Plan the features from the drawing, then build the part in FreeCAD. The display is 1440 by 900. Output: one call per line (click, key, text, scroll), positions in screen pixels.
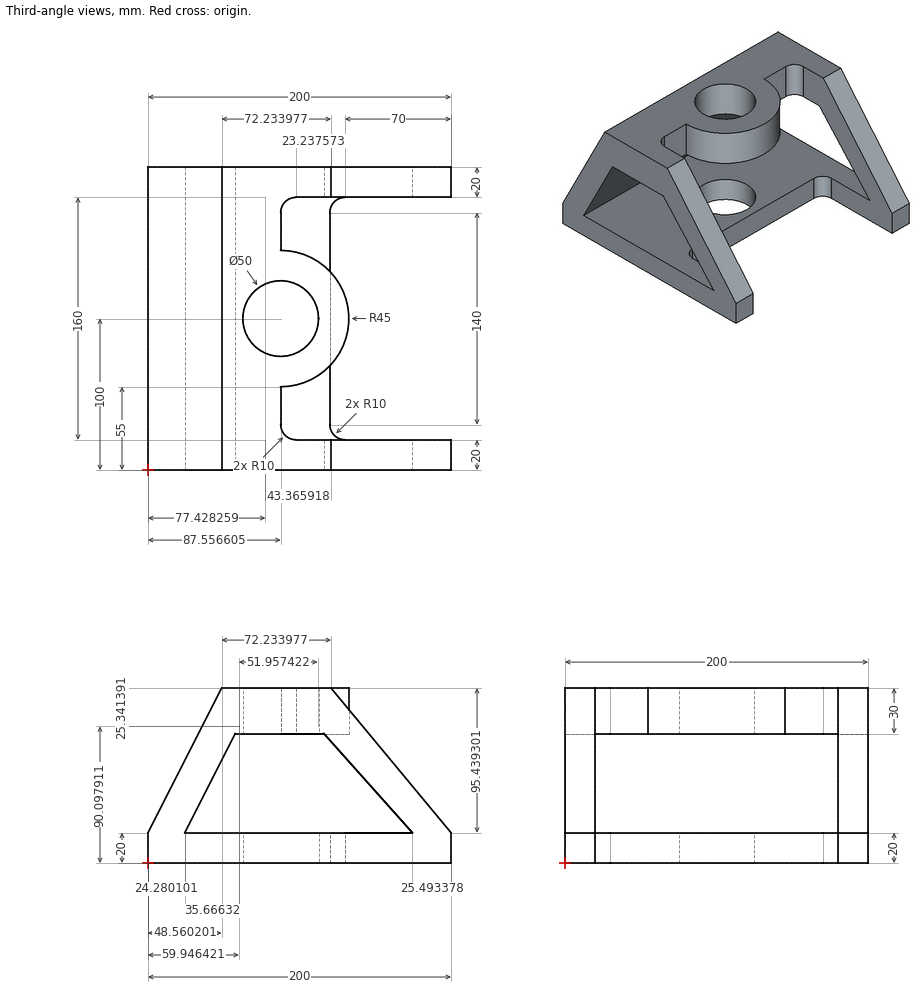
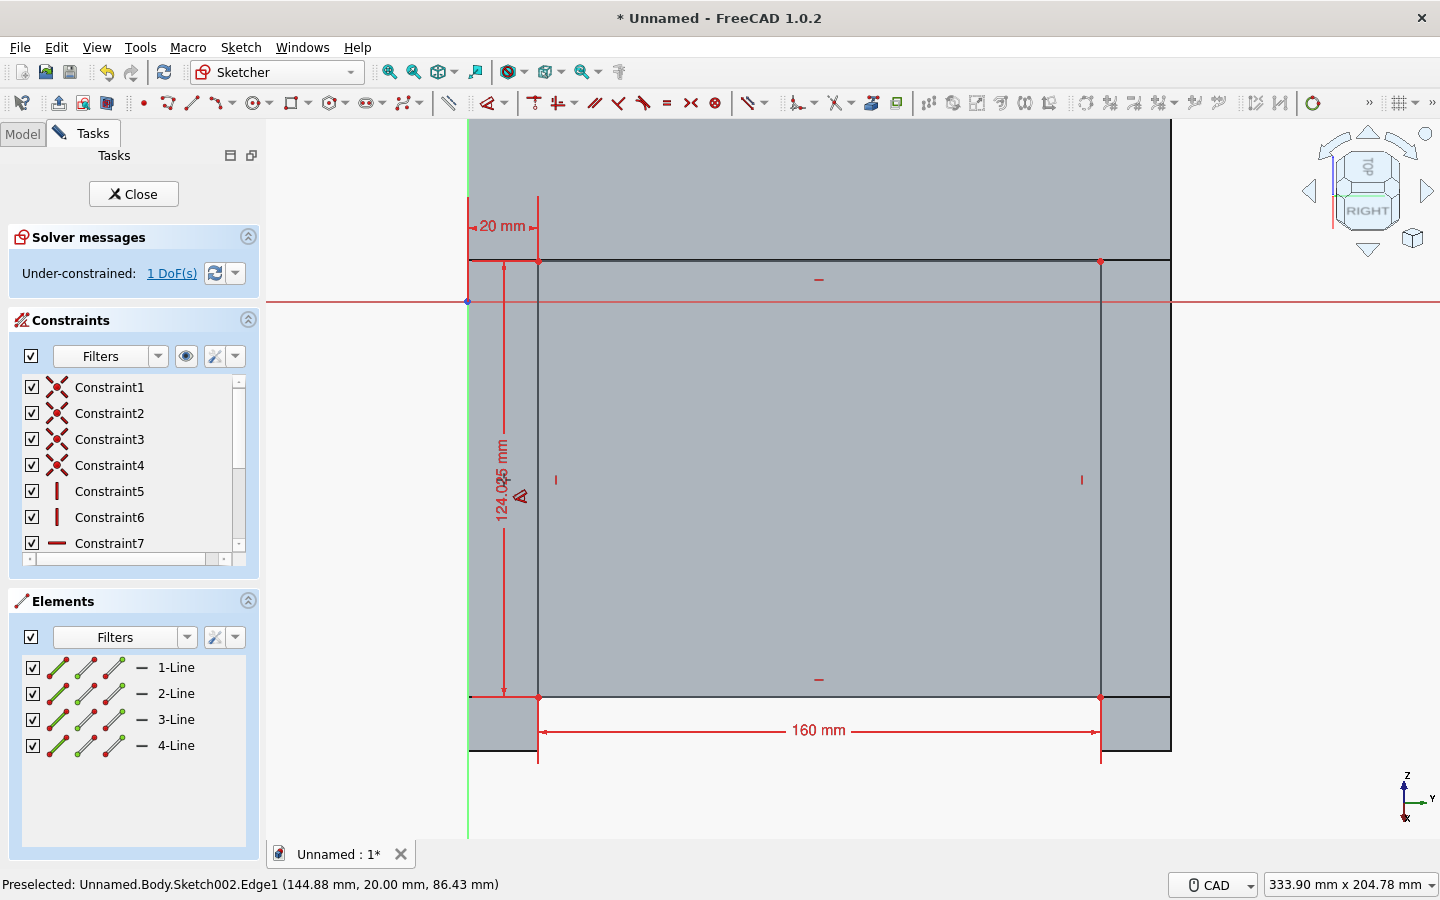
click(538, 261)
click(434, 281)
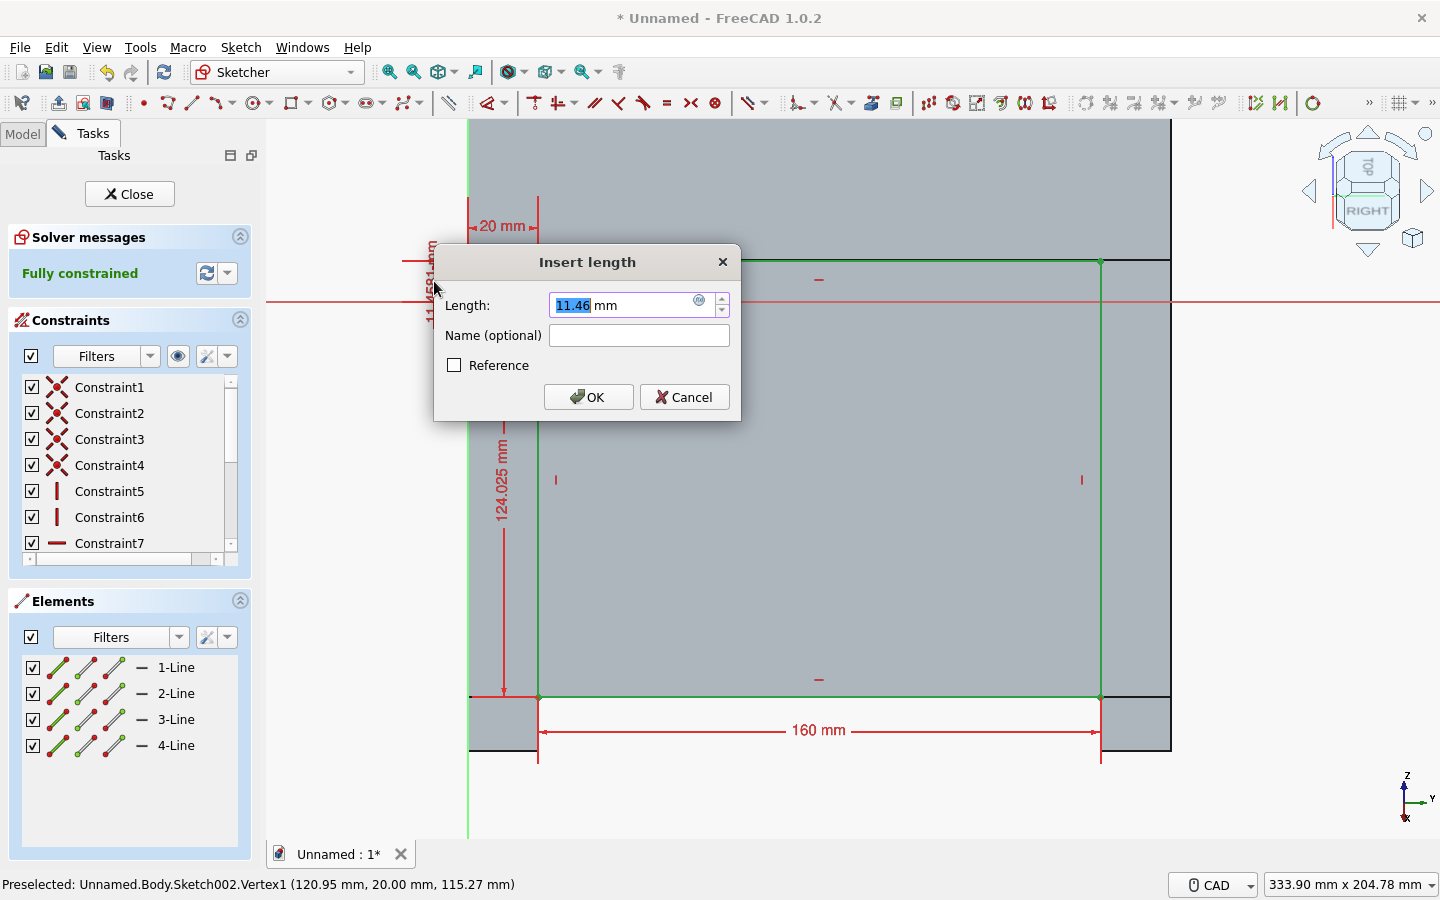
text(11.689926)
key(Return)
key(Escape)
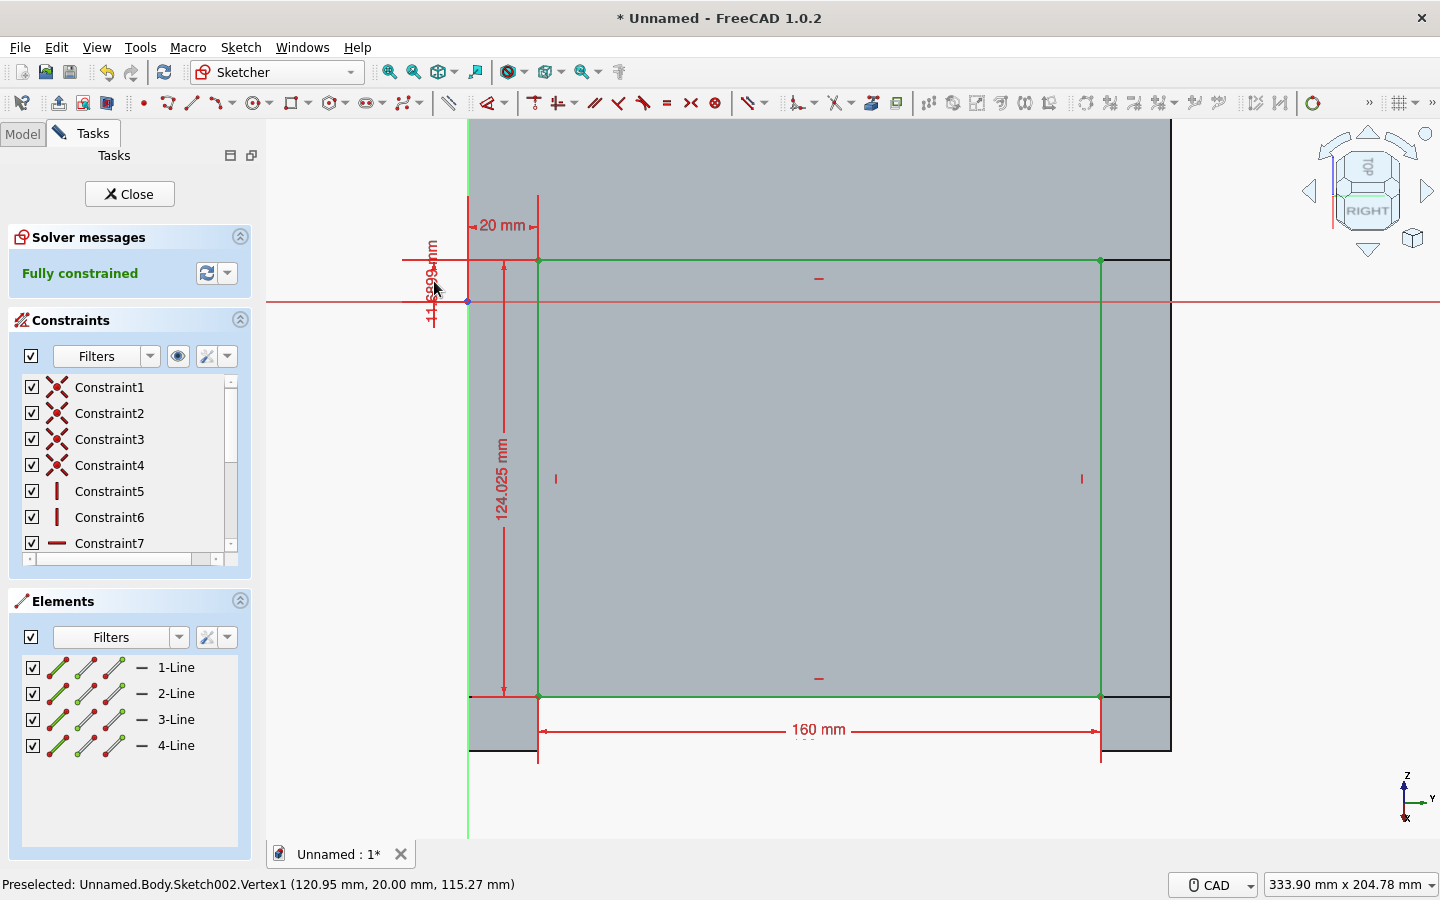
click(130, 194)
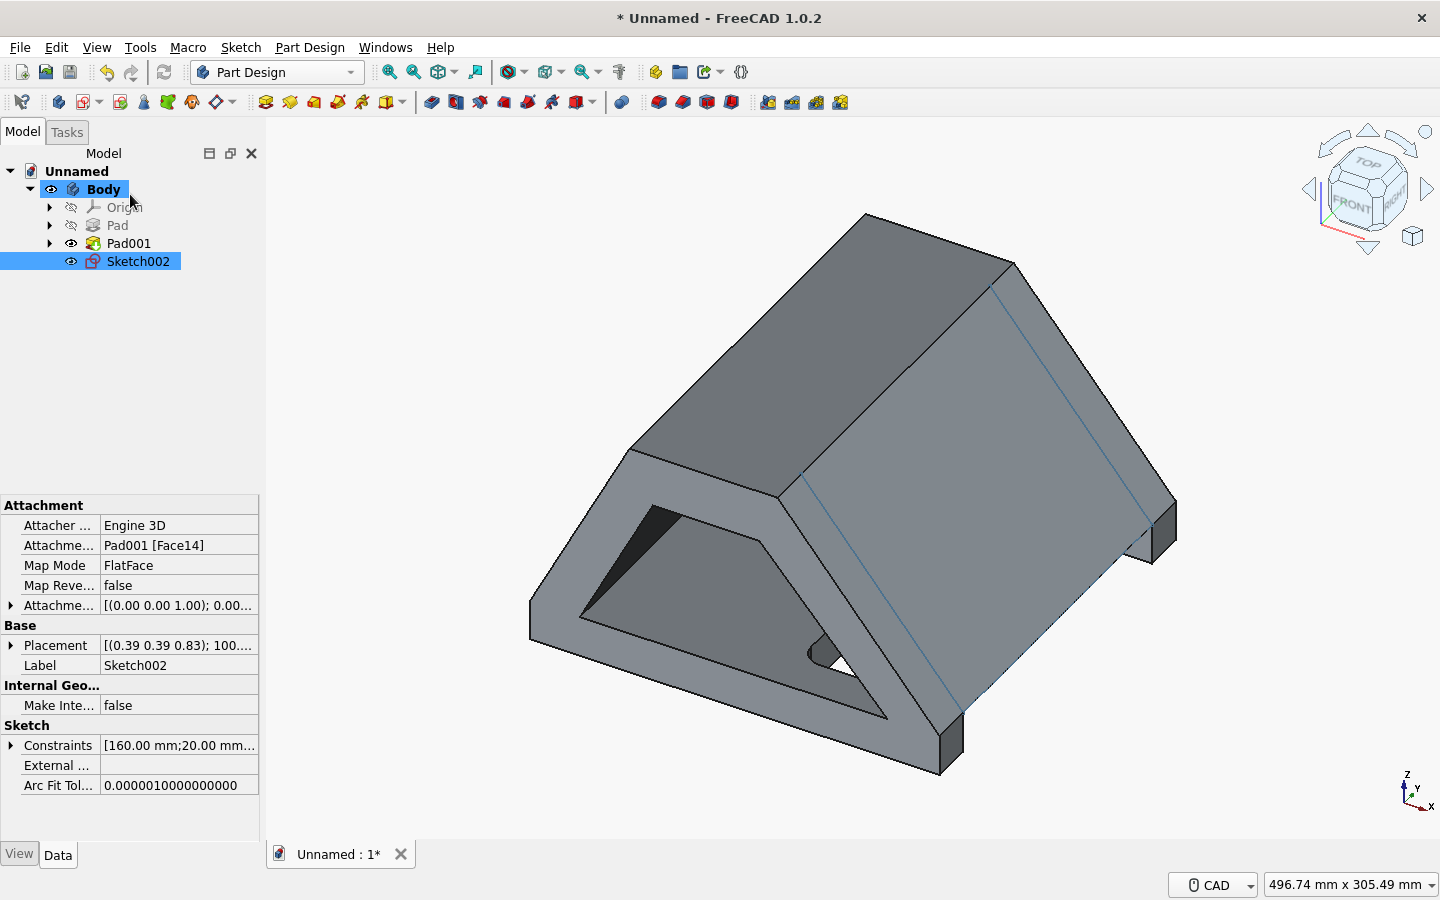
click(432, 102)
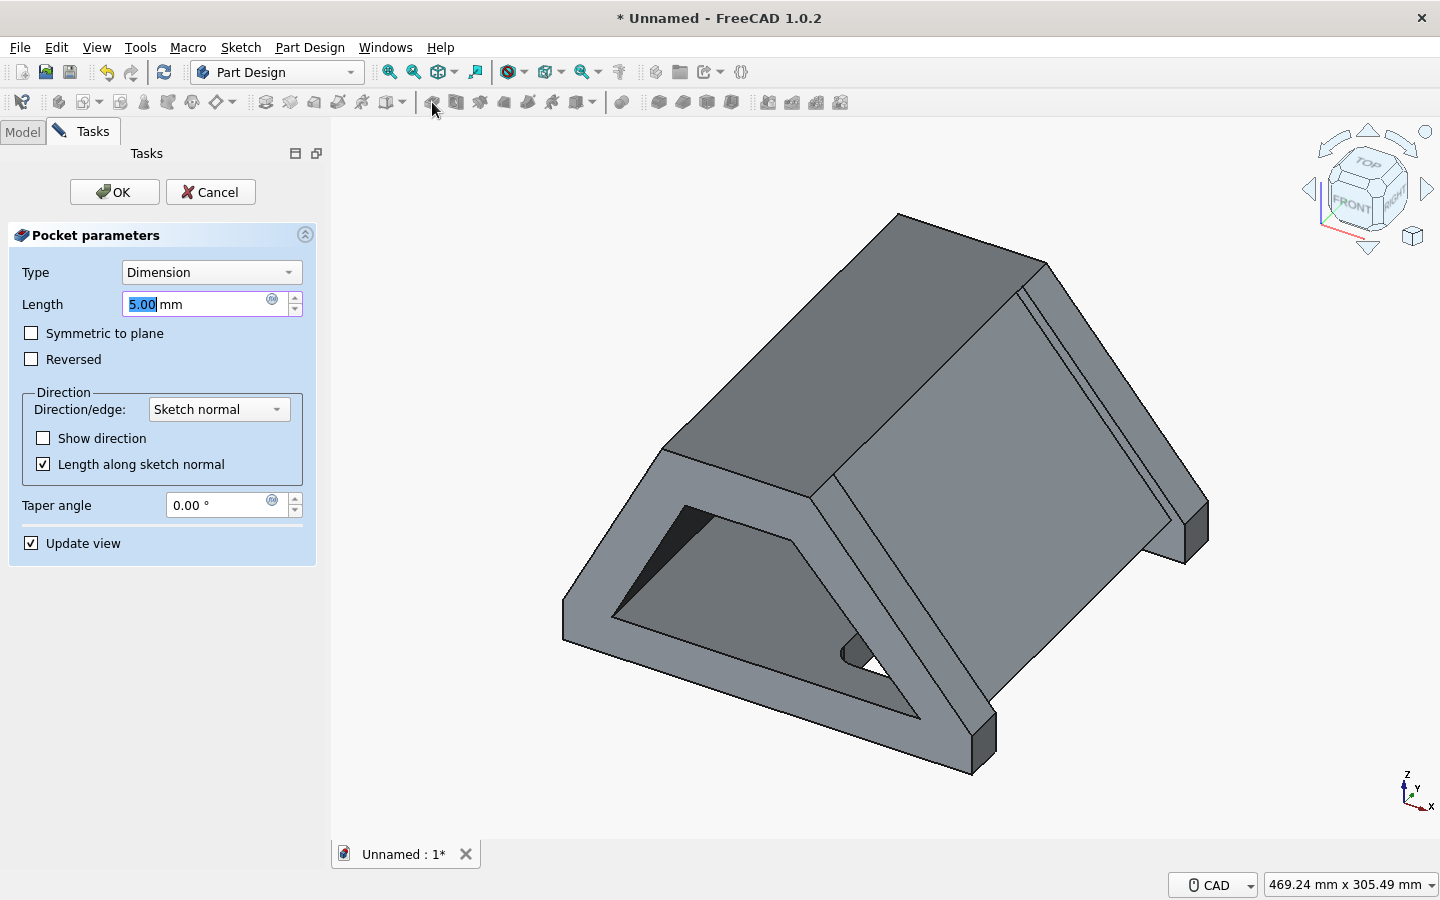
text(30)
key(Tab)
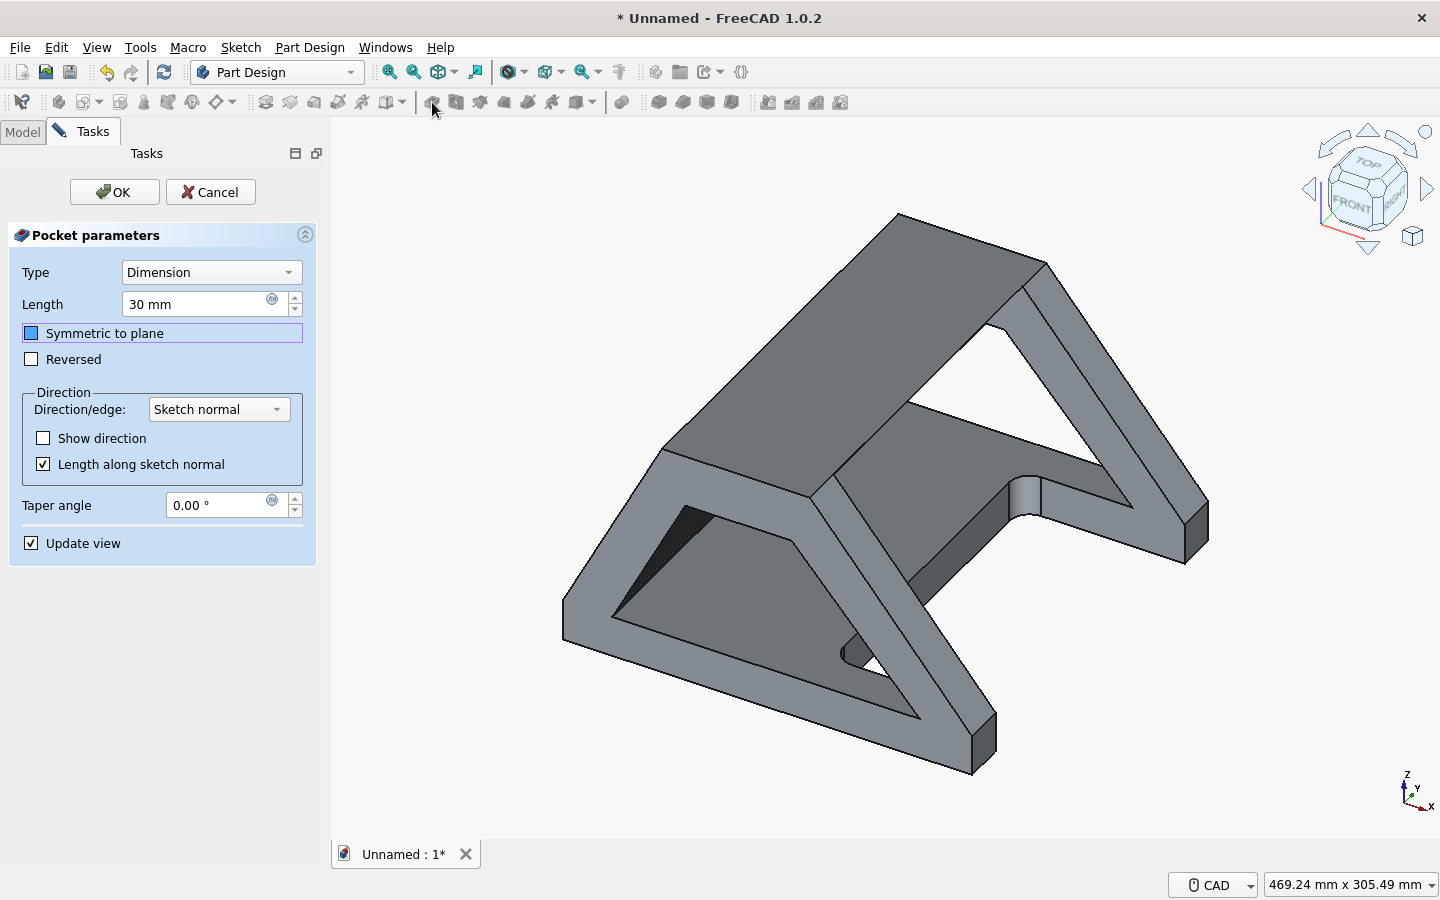
click(115, 192)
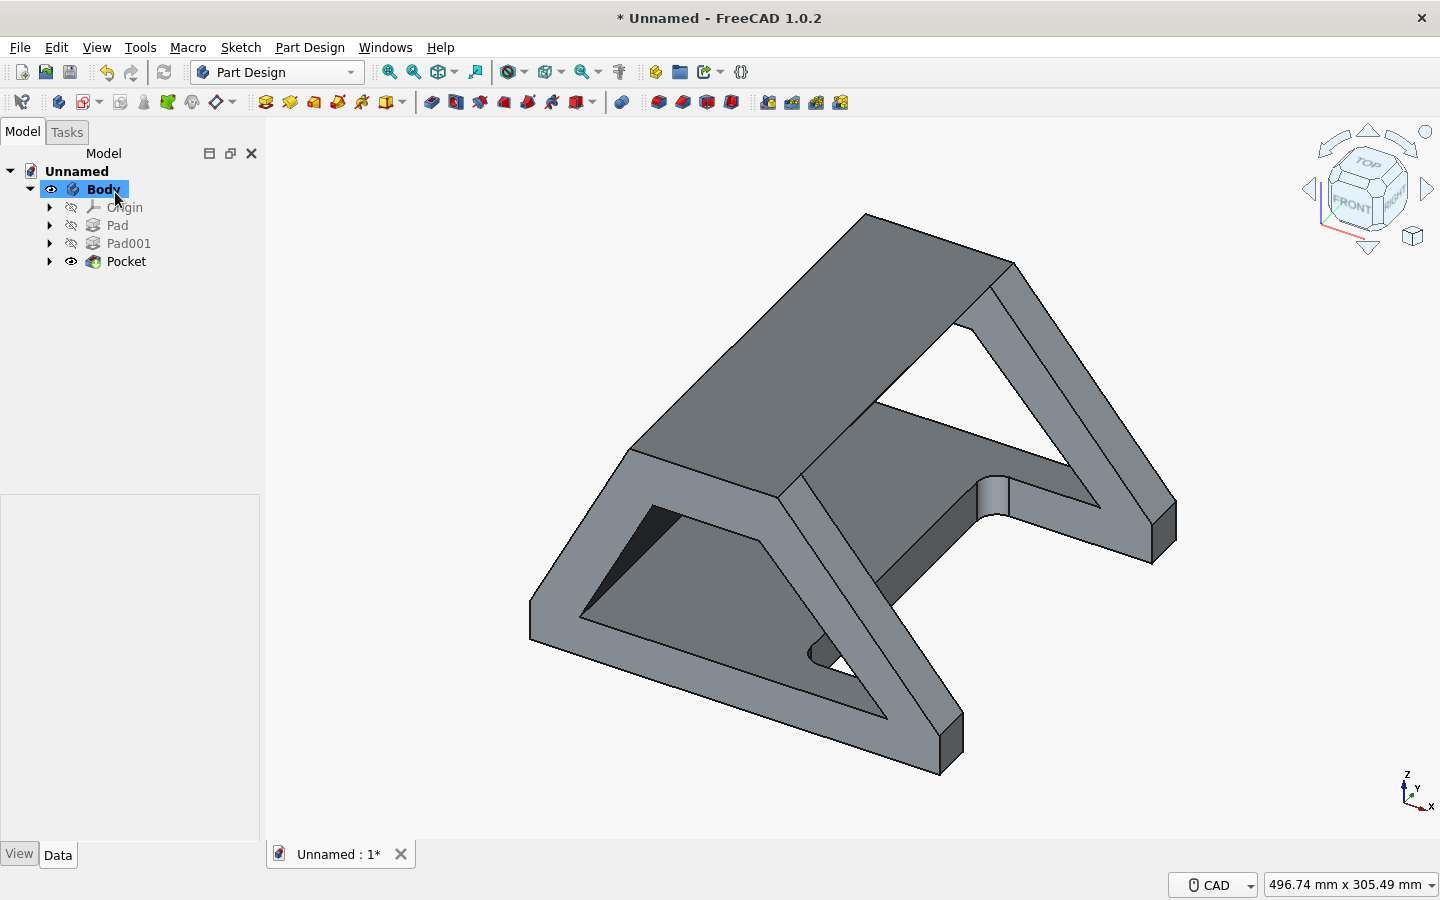
click(889, 288)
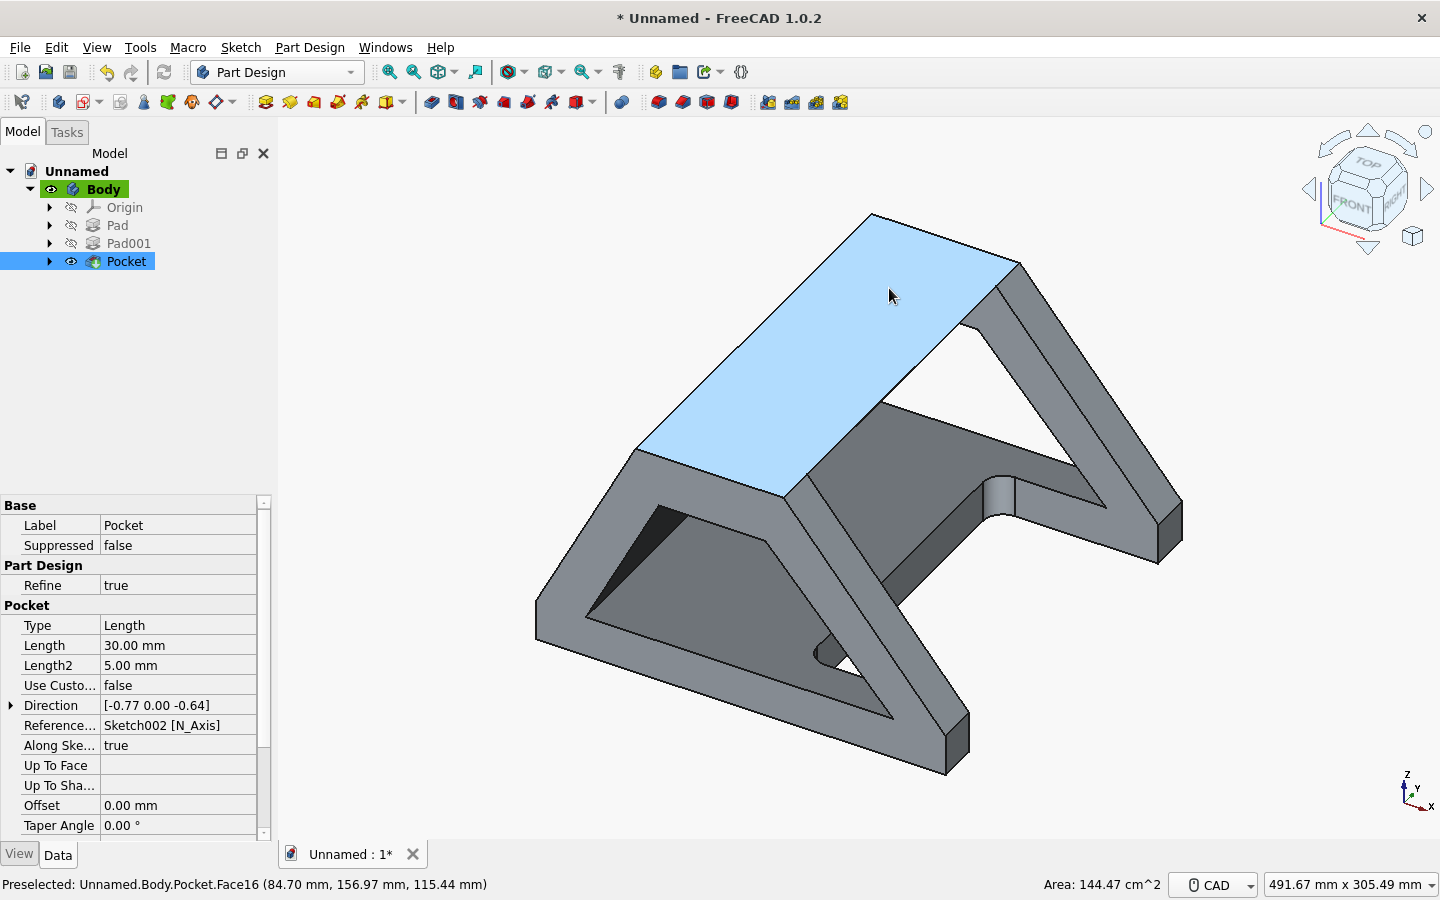
click(84, 102)